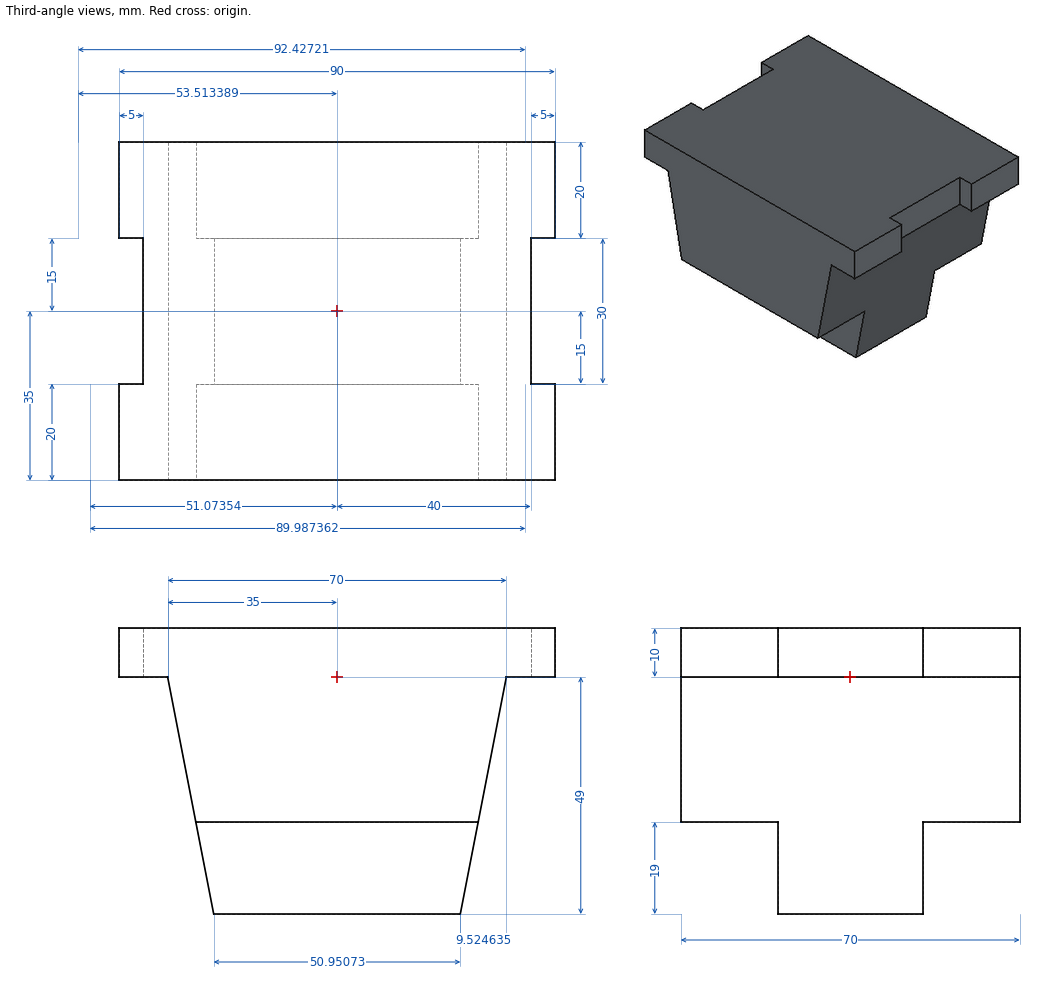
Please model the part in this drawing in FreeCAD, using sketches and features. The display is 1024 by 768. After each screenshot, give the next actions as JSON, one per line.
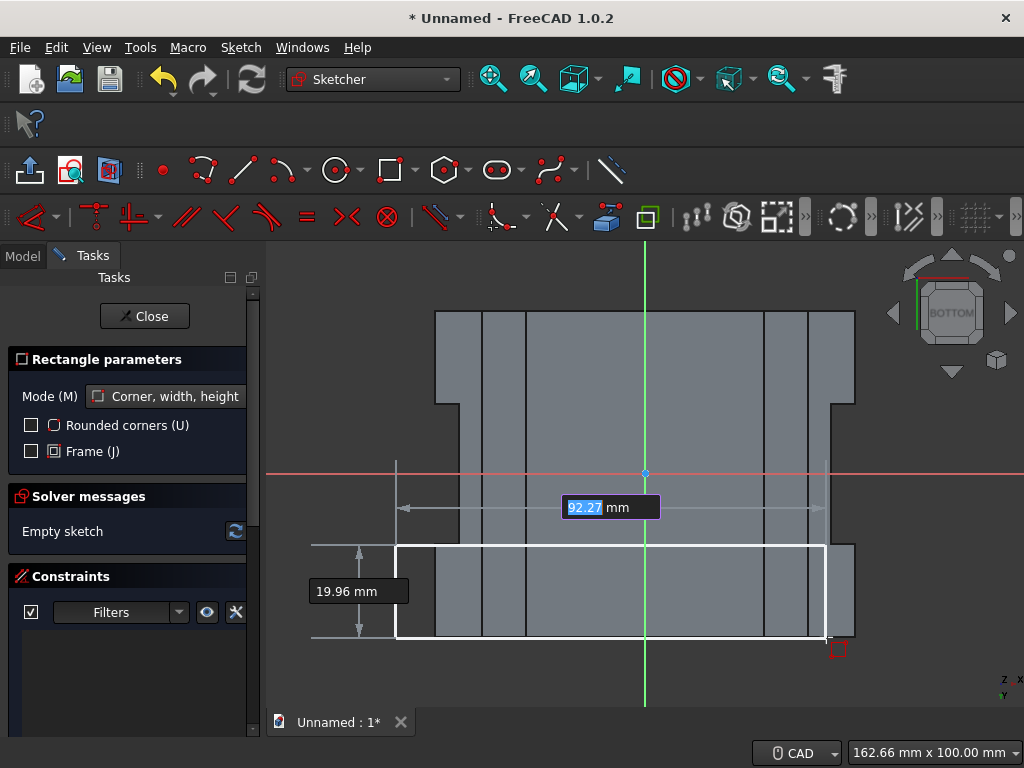
{"action": "type", "text": "92.42721"}
{"action": "key", "text": "Tab"}
{"action": "type", "text": "20"}
{"action": "key", "text": "Return"}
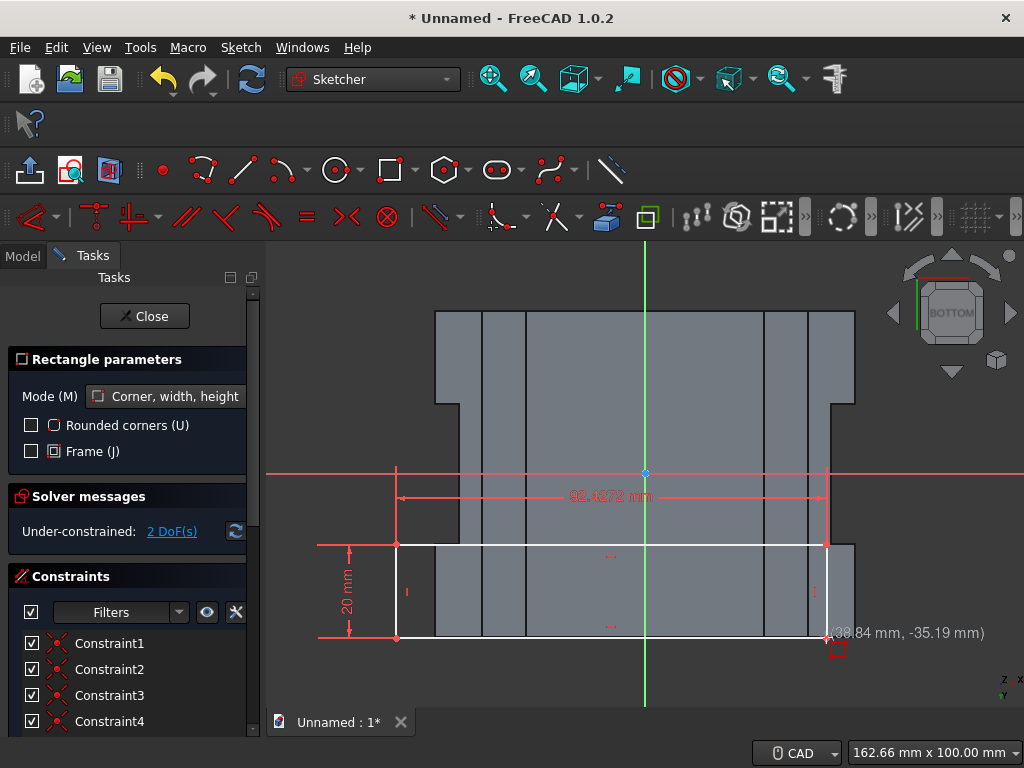
{"action": "left_click", "coordinate": [407, 311]}
{"action": "mouse_move", "coordinate": [826, 404]}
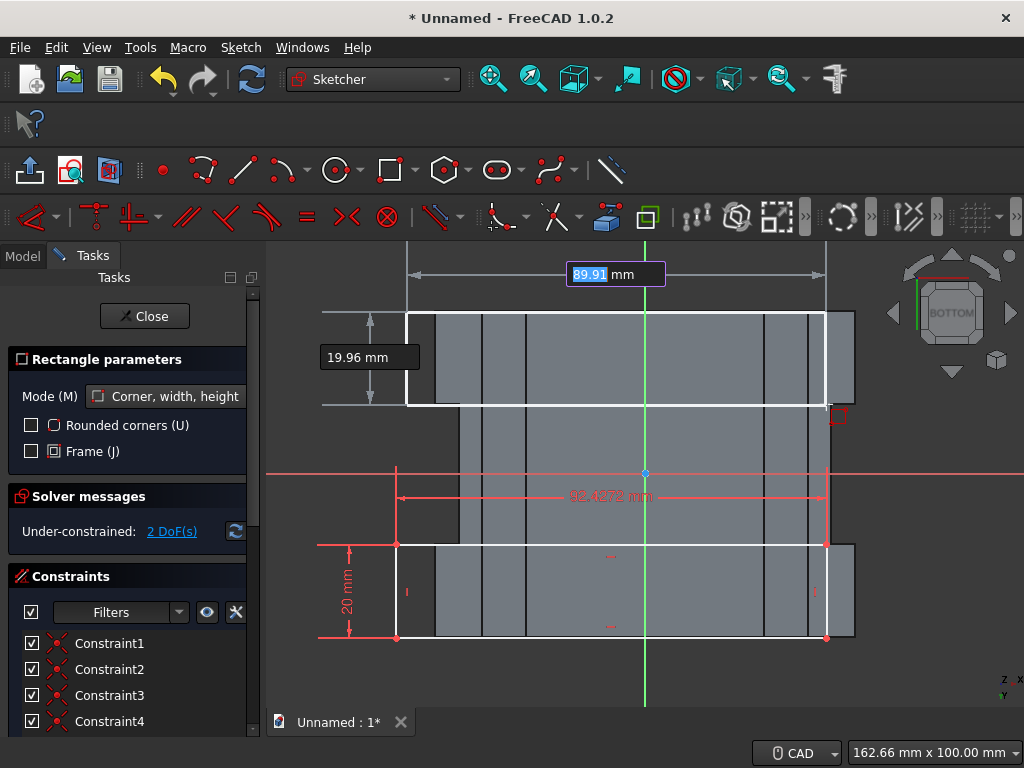
{"action": "type", "text": "89.987362"}
{"action": "key", "text": "Tab"}
{"action": "type", "text": "20"}
{"action": "key", "text": "Return"}
{"action": "key", "text": "Escape"}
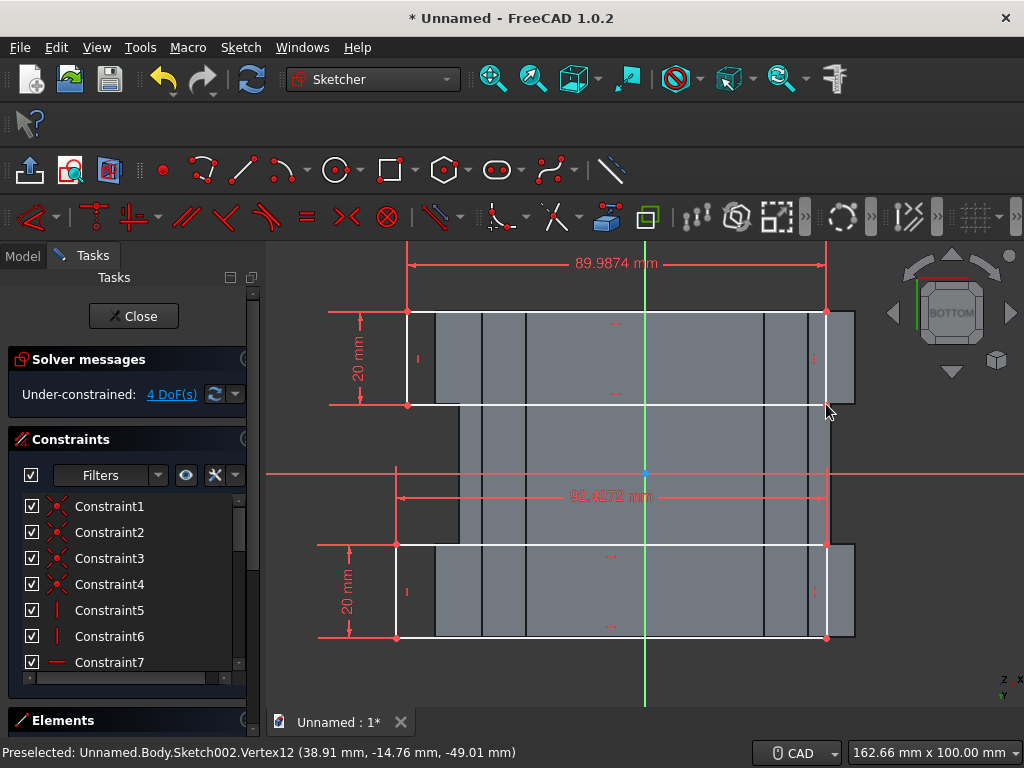
{"action": "left_click", "coordinate": [32, 218]}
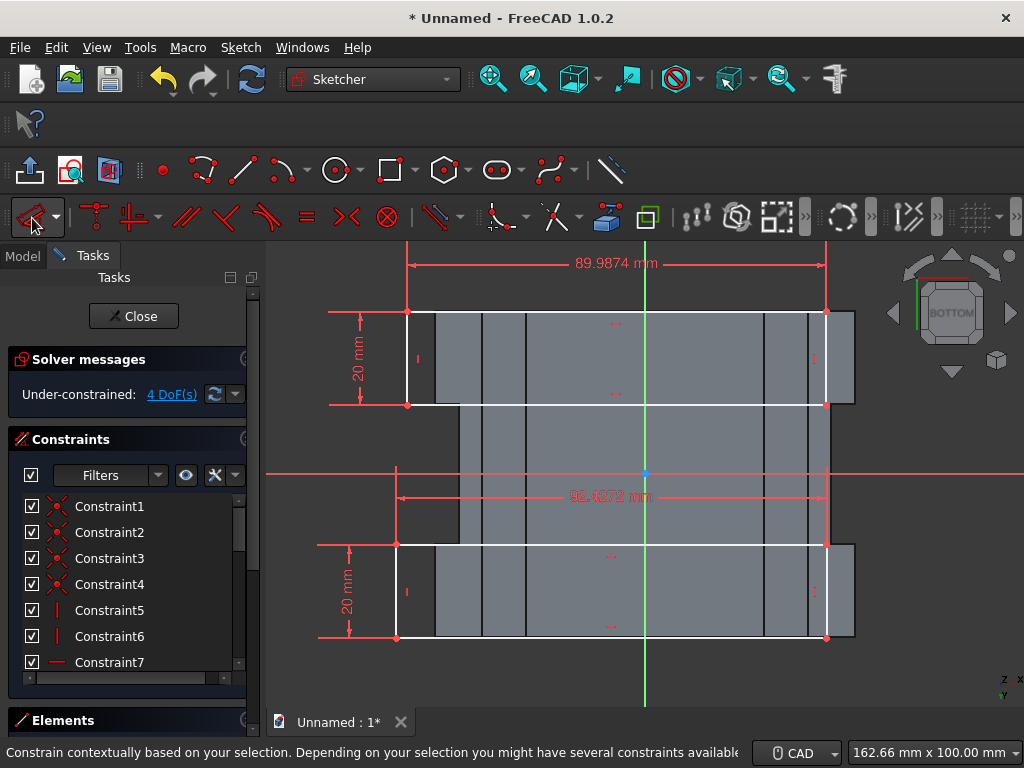
{"action": "left_click", "coordinate": [396, 545]}
{"action": "left_click", "coordinate": [362, 510]}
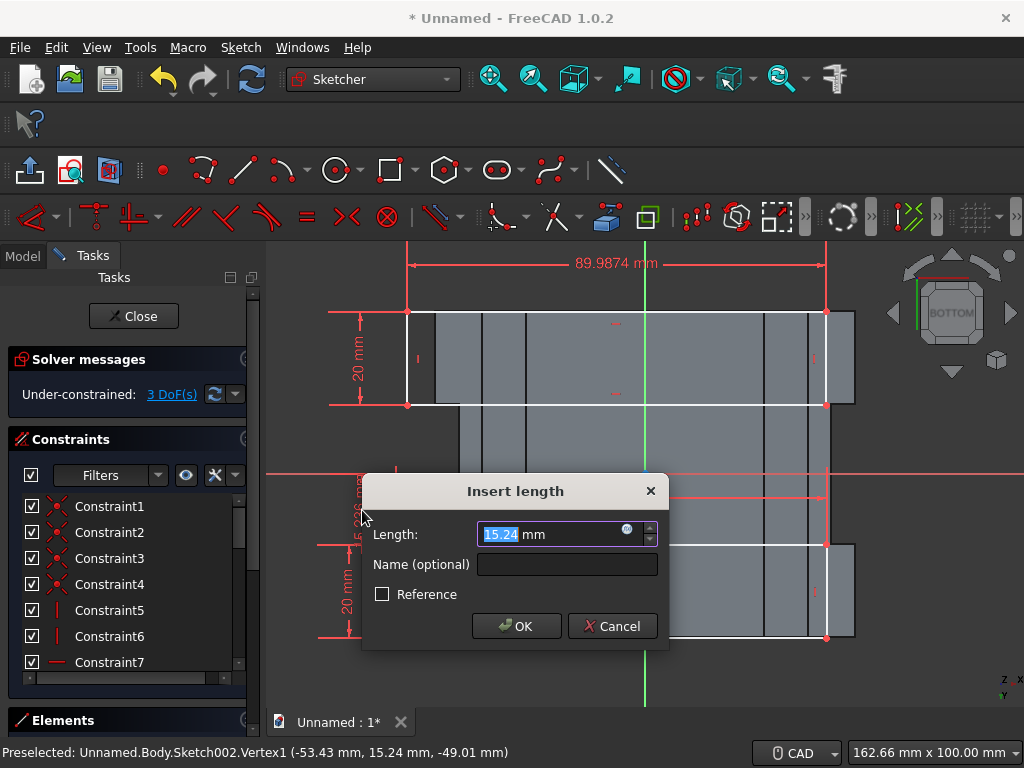
{"action": "type", "text": "15"}
{"action": "key", "text": "Return"}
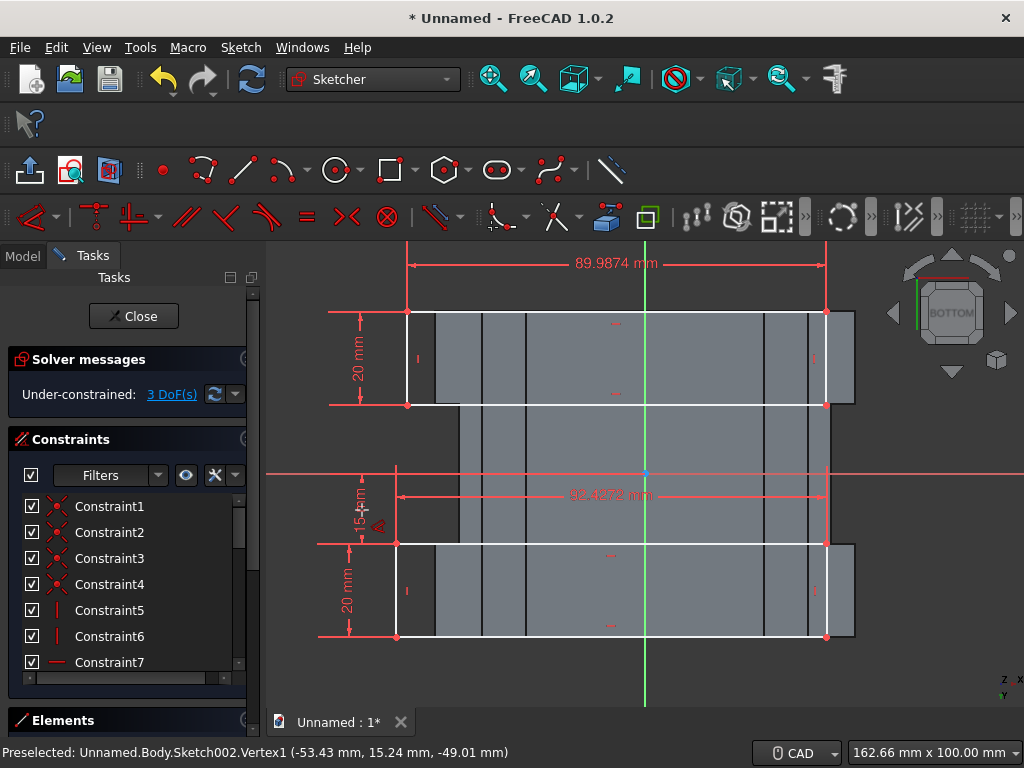
{"action": "left_click", "coordinate": [407, 312]}
{"action": "left_click", "coordinate": [373, 393]}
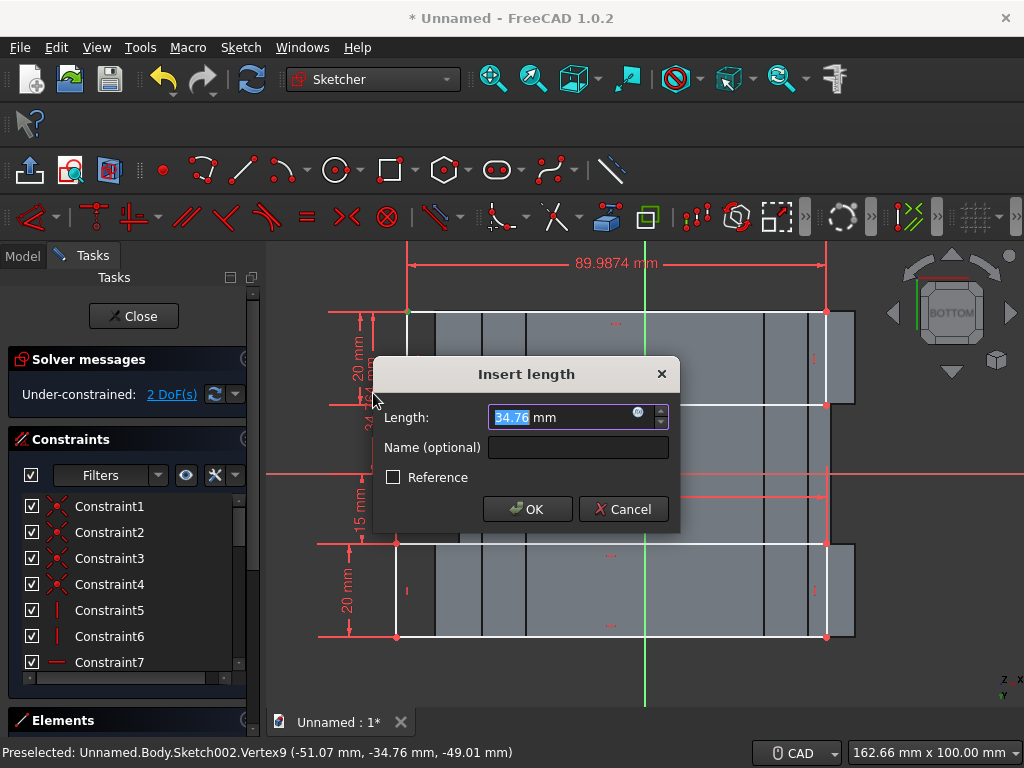
{"action": "type", "text": "35"}
{"action": "key", "text": "Return"}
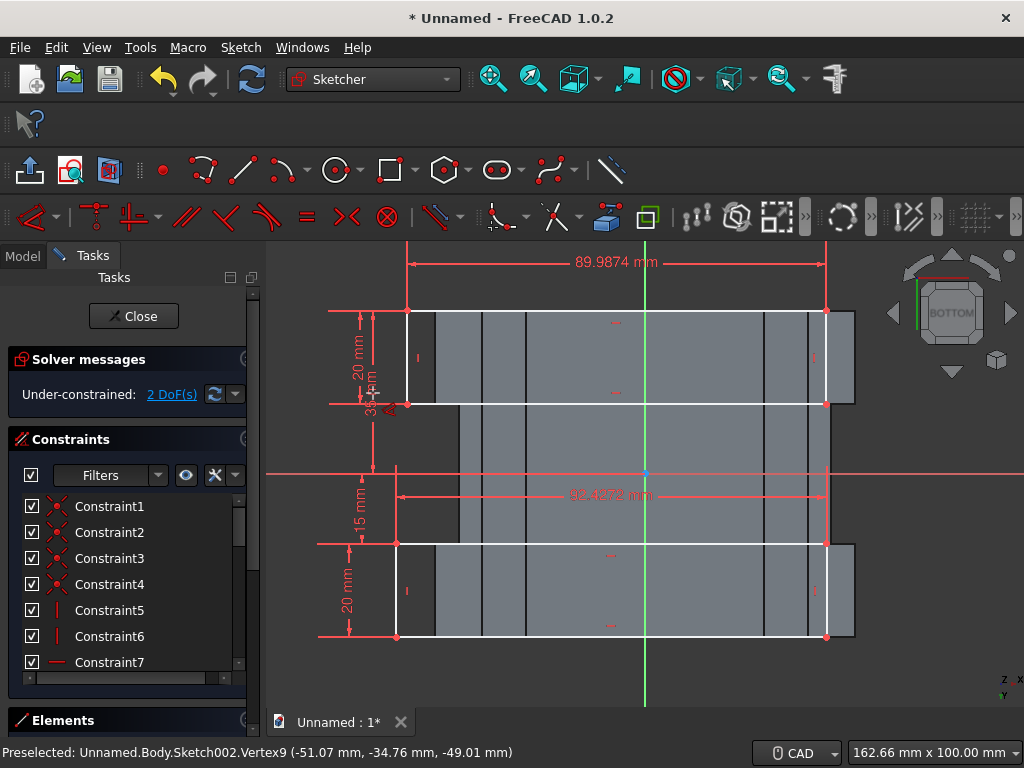
{"action": "left_click", "coordinate": [407, 311]}
{"action": "left_click", "coordinate": [526, 277]}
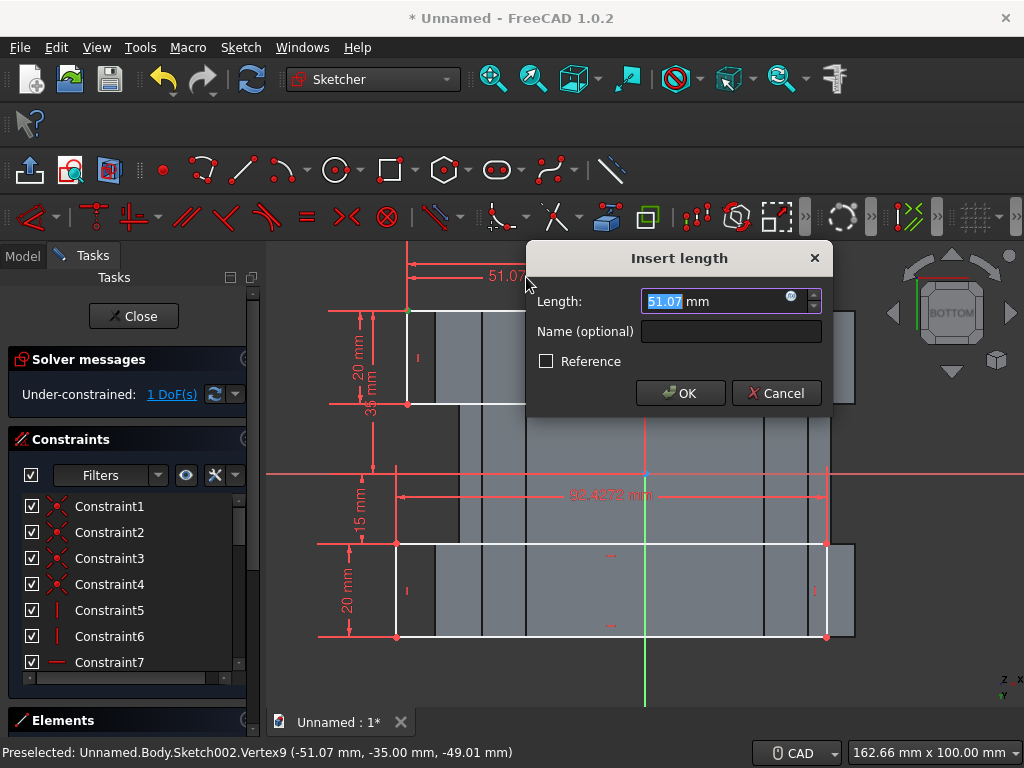
{"action": "type", "text": "51.07354"}
{"action": "key", "text": "Return"}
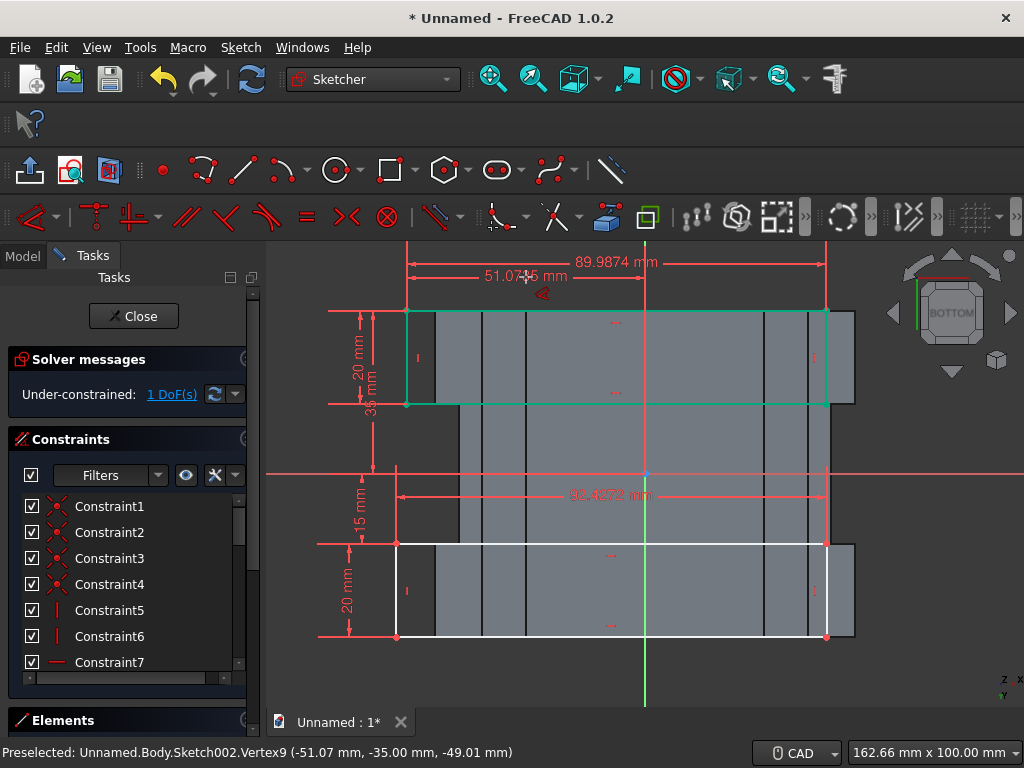
{"action": "left_click", "coordinate": [396, 544]}
{"action": "left_click", "coordinate": [520, 578]}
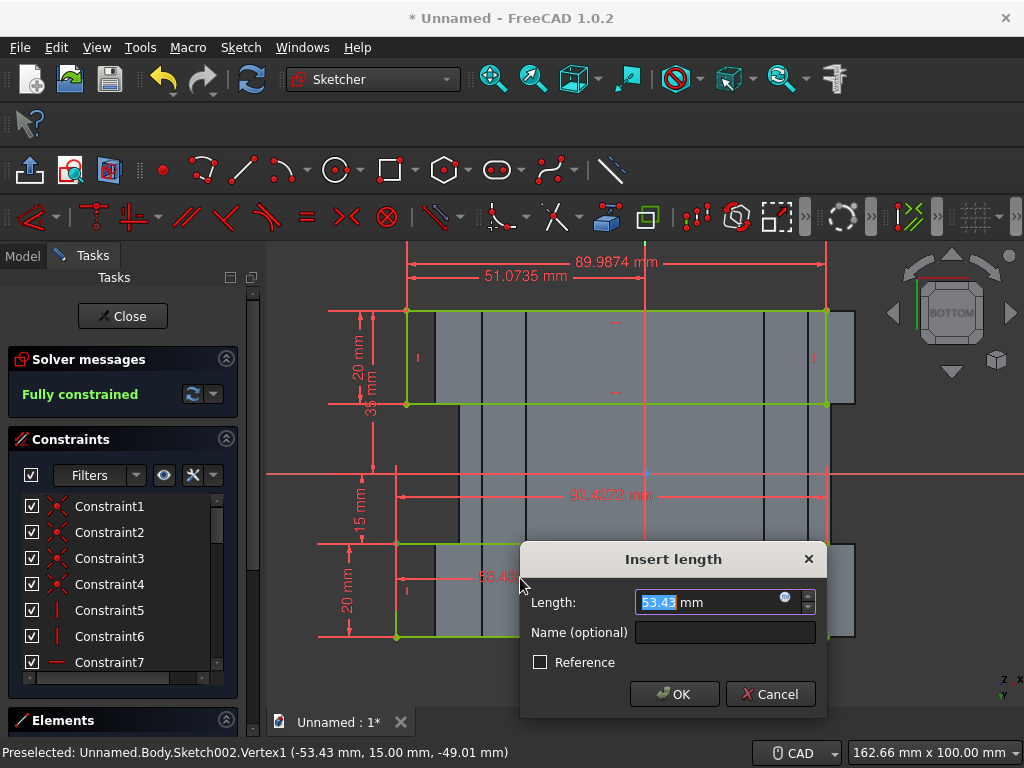
{"action": "type", "text": "53.513389"}
{"action": "key", "text": "Return"}
{"action": "key", "text": "Escape"}